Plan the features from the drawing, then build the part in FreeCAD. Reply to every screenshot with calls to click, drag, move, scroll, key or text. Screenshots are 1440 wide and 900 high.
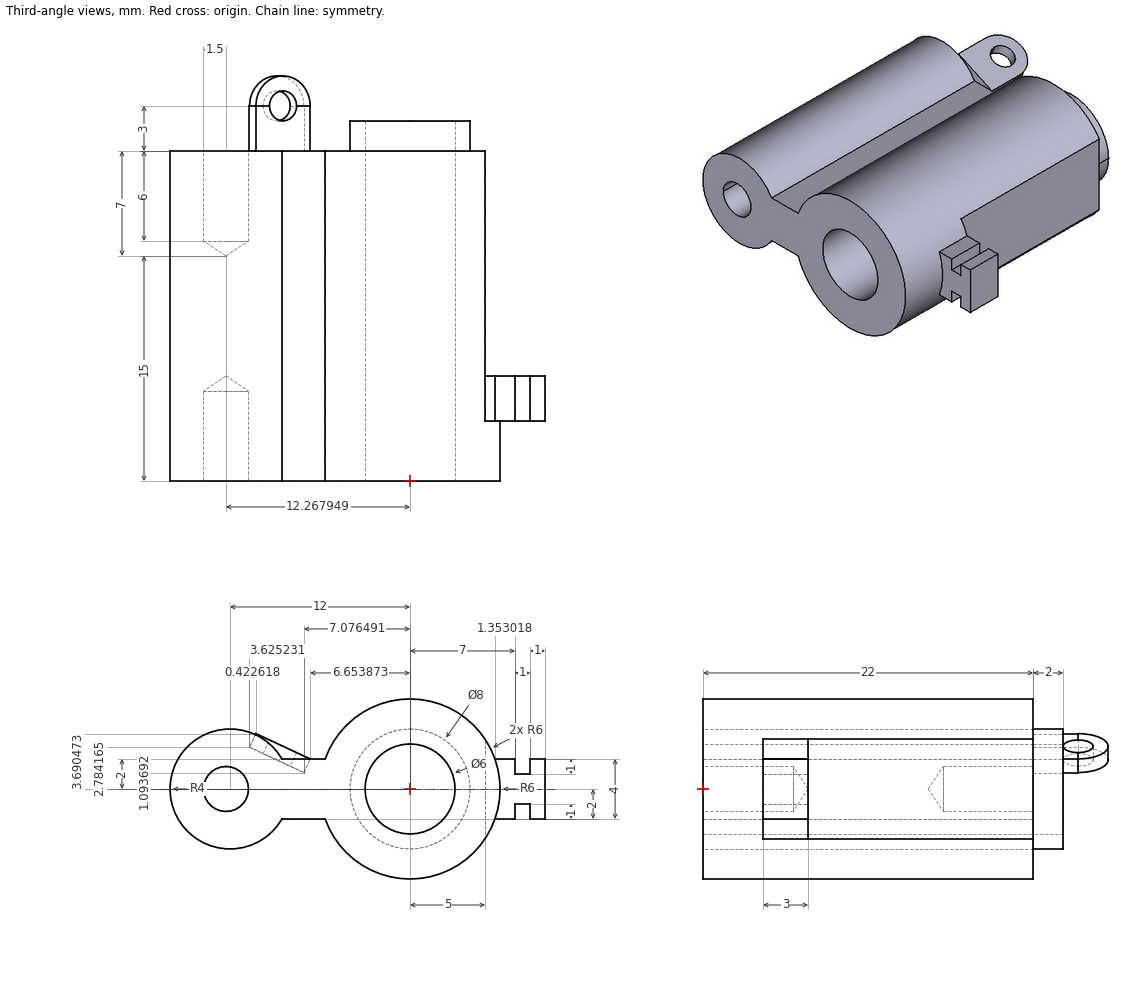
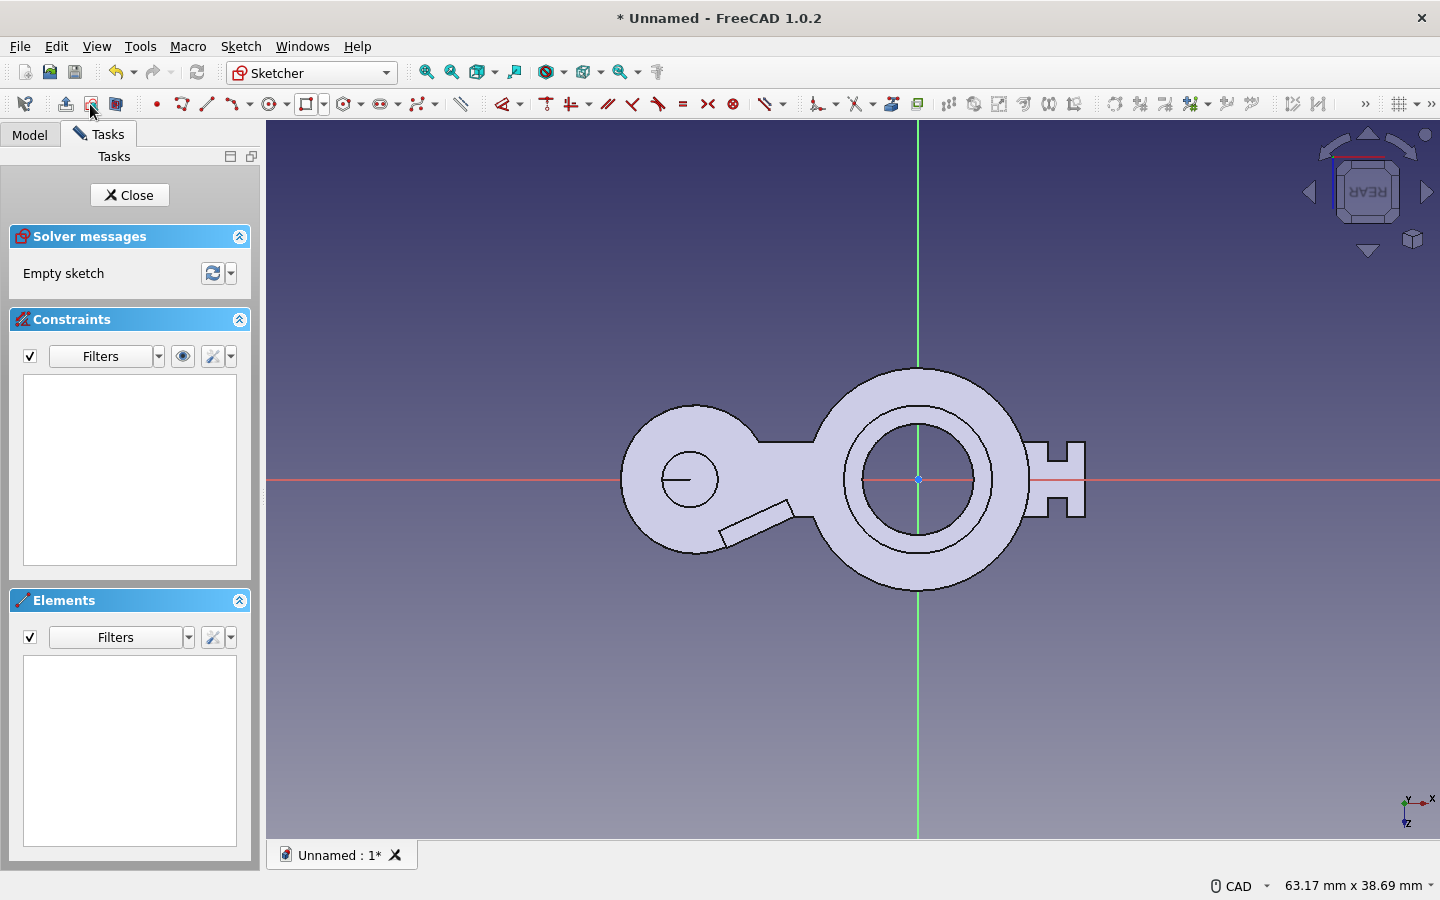
click(116, 104)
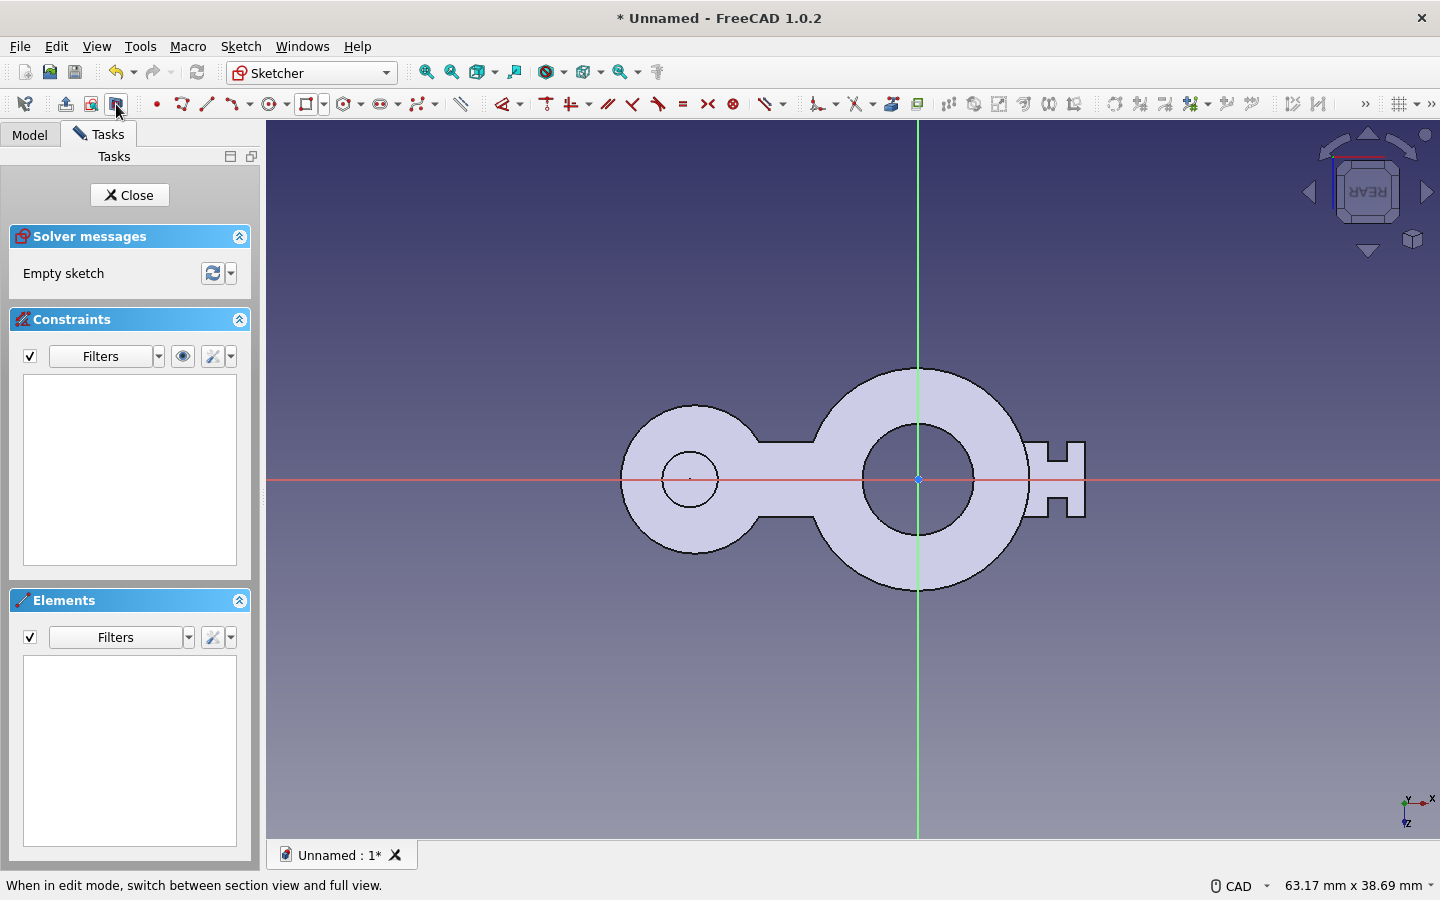
scroll(1036, 479, up, 7)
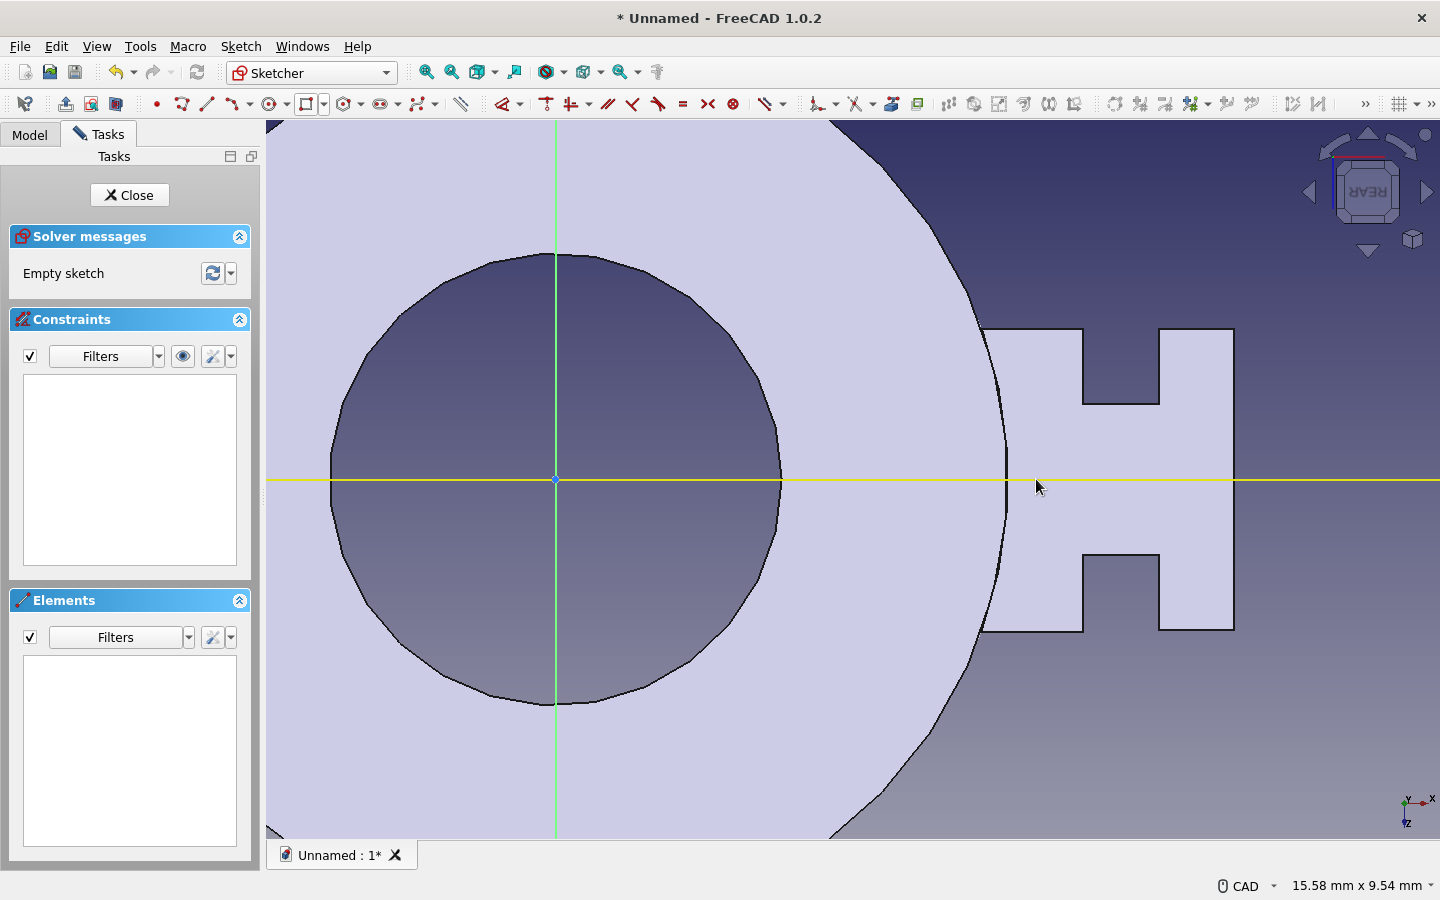
click(207, 104)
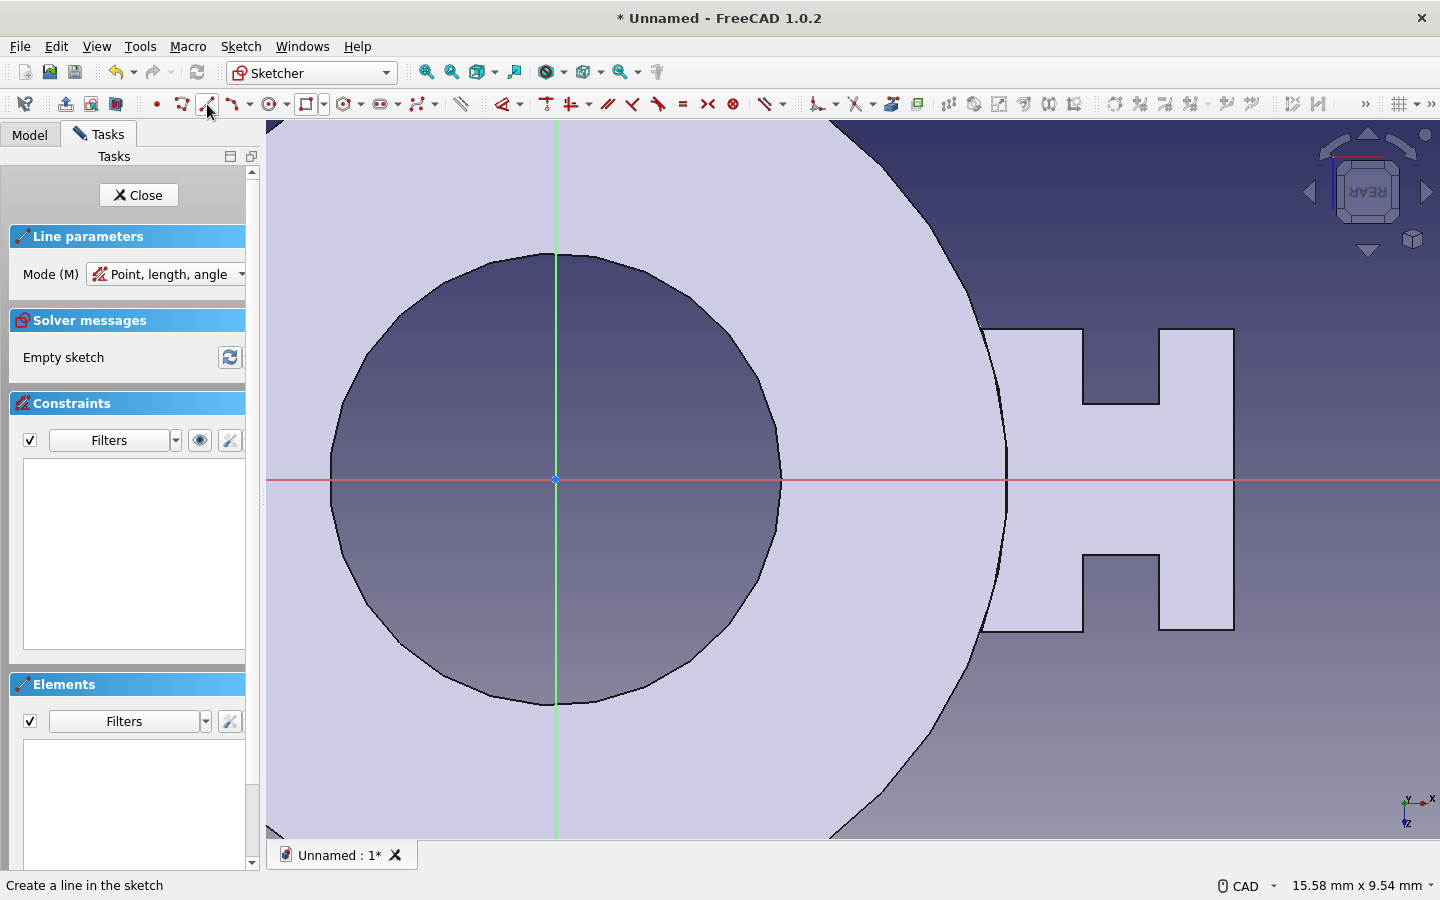
click(932, 230)
click(932, 729)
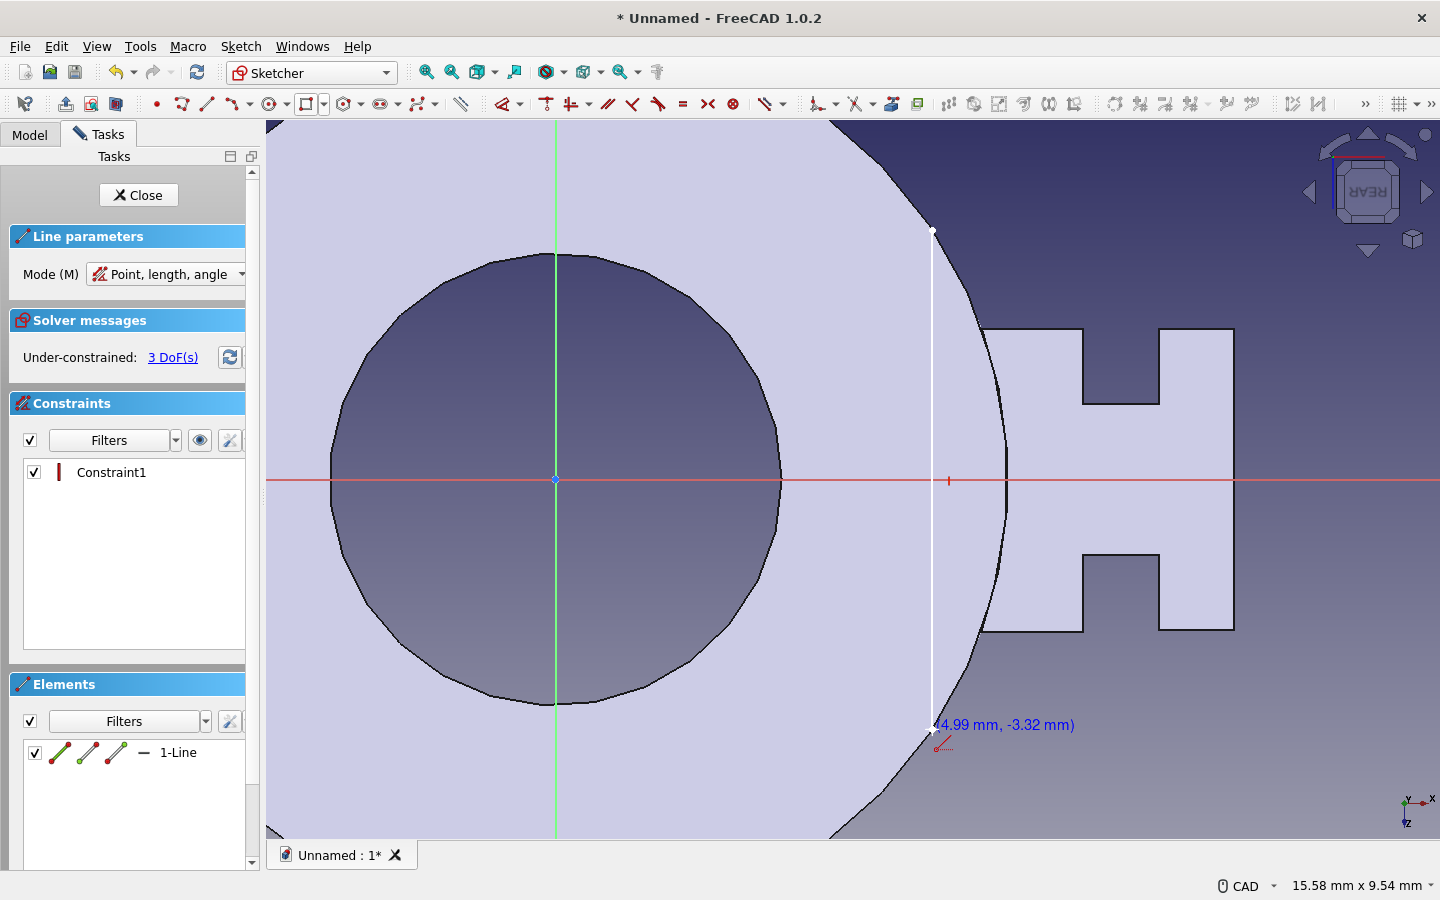
click(232, 104)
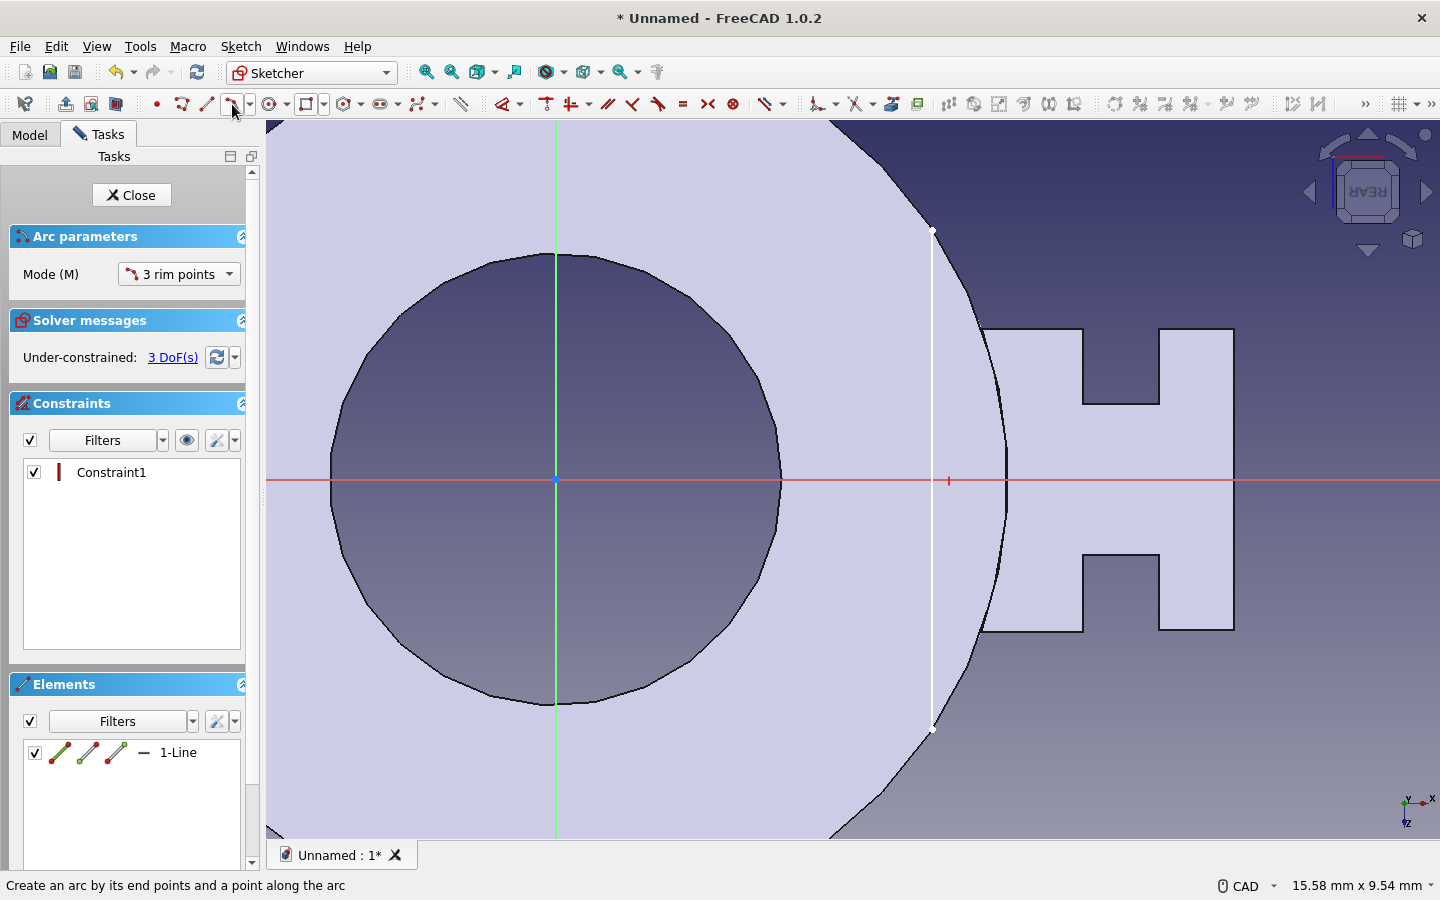
click(932, 730)
click(932, 231)
click(1005, 532)
key(Escape)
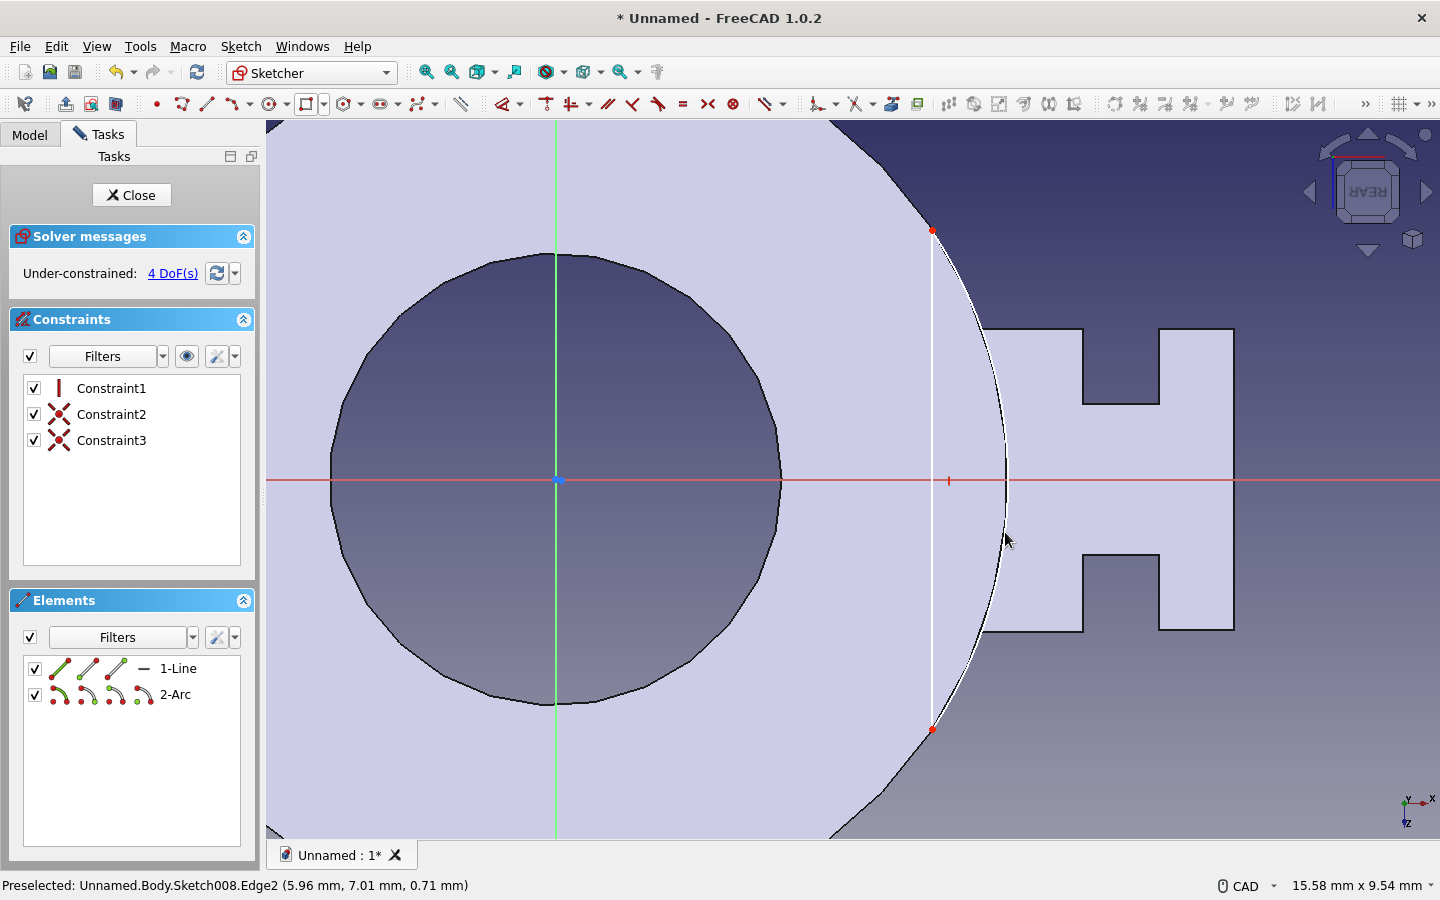
drag(546, 469, 571, 490)